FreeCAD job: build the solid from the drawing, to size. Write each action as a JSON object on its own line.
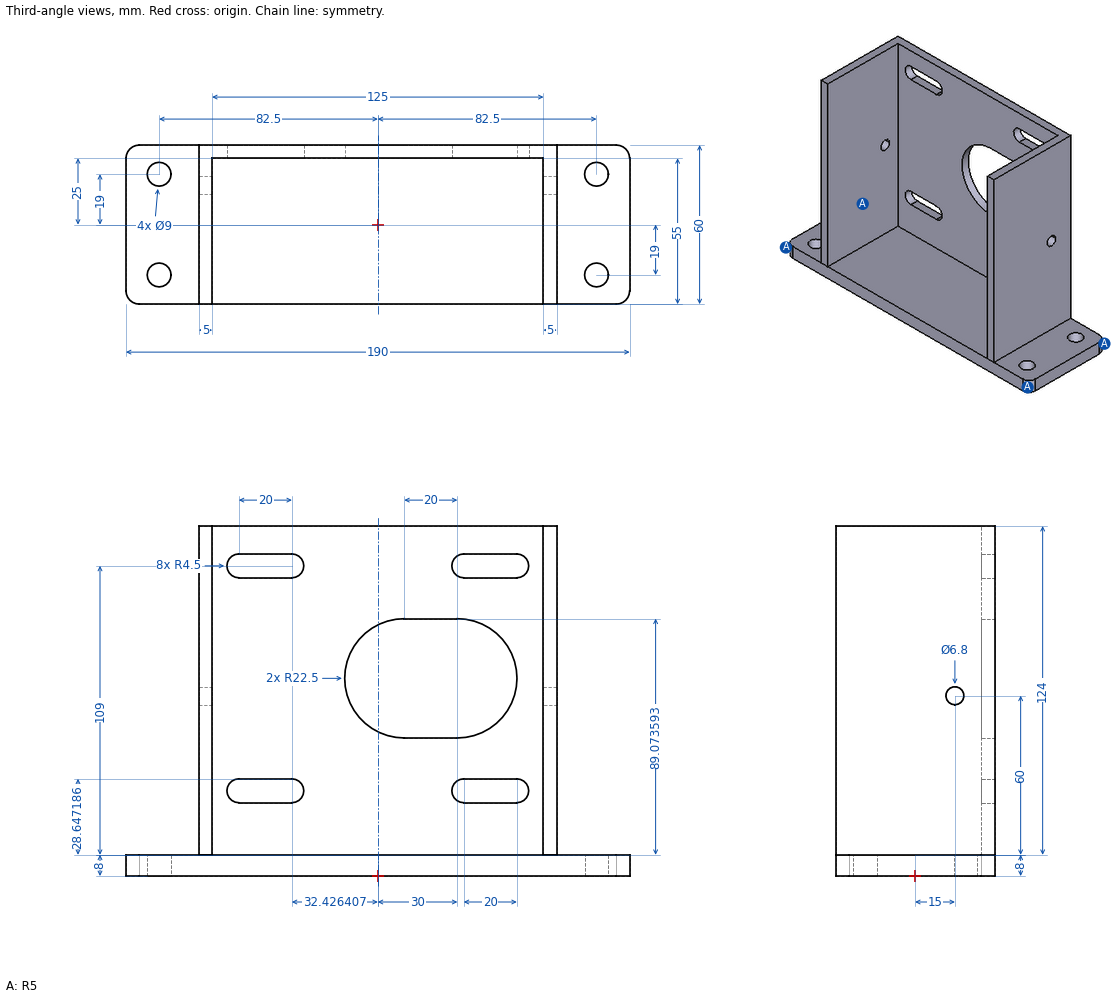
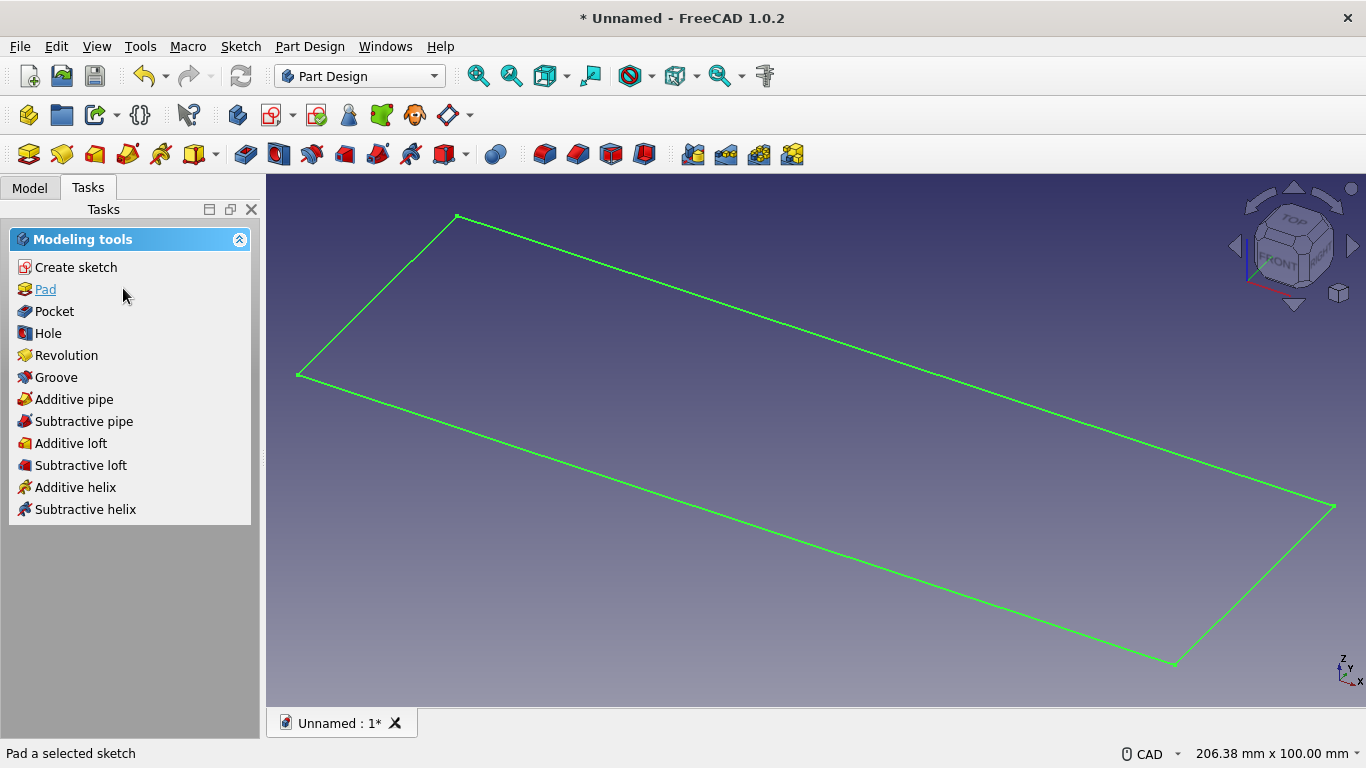
{"action": "left_click", "coordinate": [29, 154]}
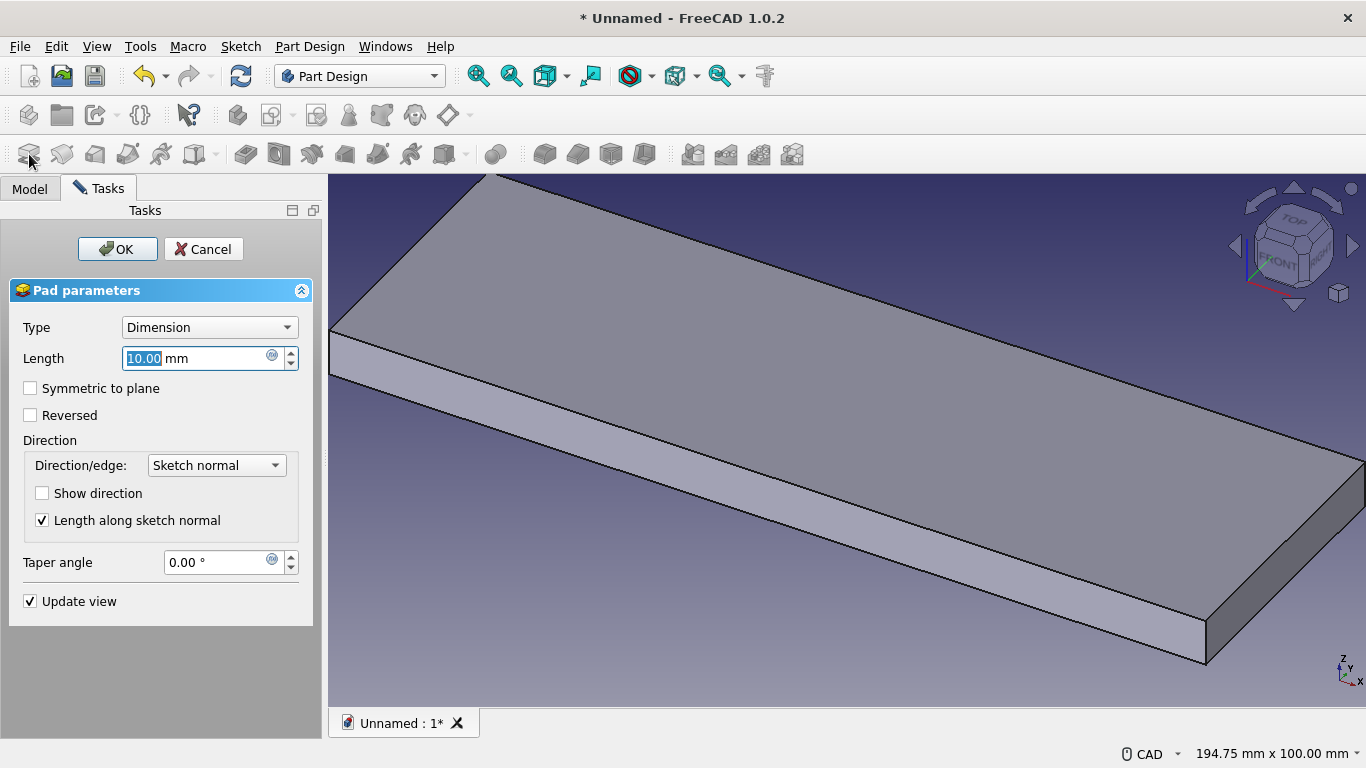
{"action": "type", "text": "8"}
{"action": "key", "text": "Tab"}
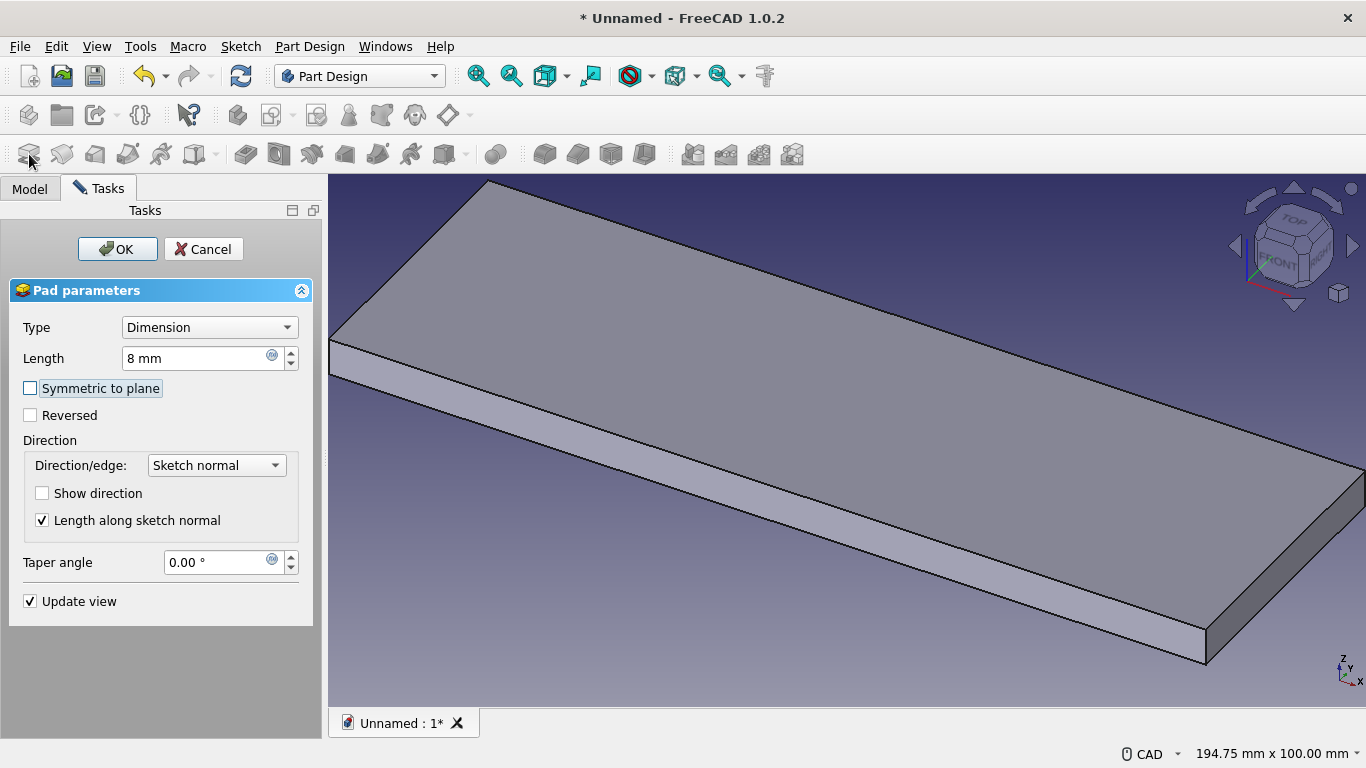
{"action": "left_click", "coordinate": [118, 249]}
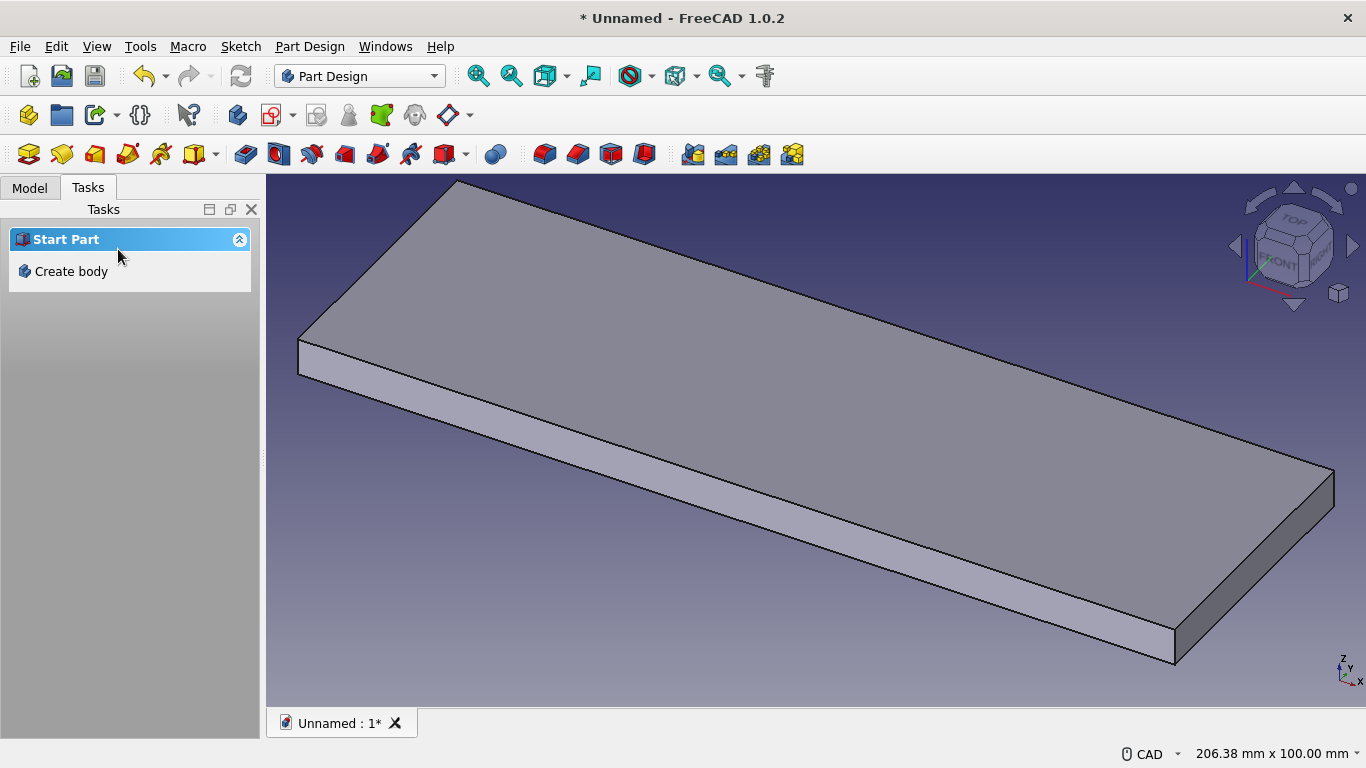
{"action": "left_click", "coordinate": [1067, 487]}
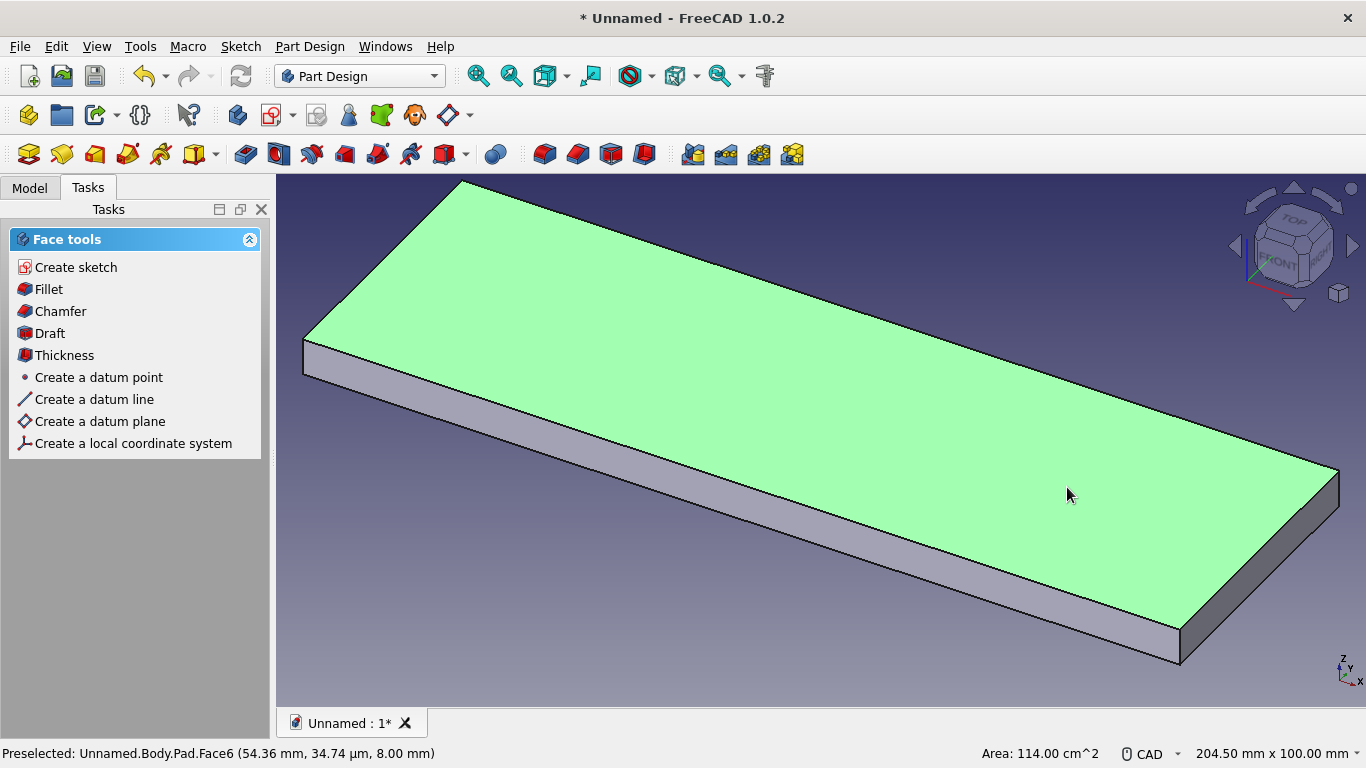
{"action": "left_click", "coordinate": [270, 116]}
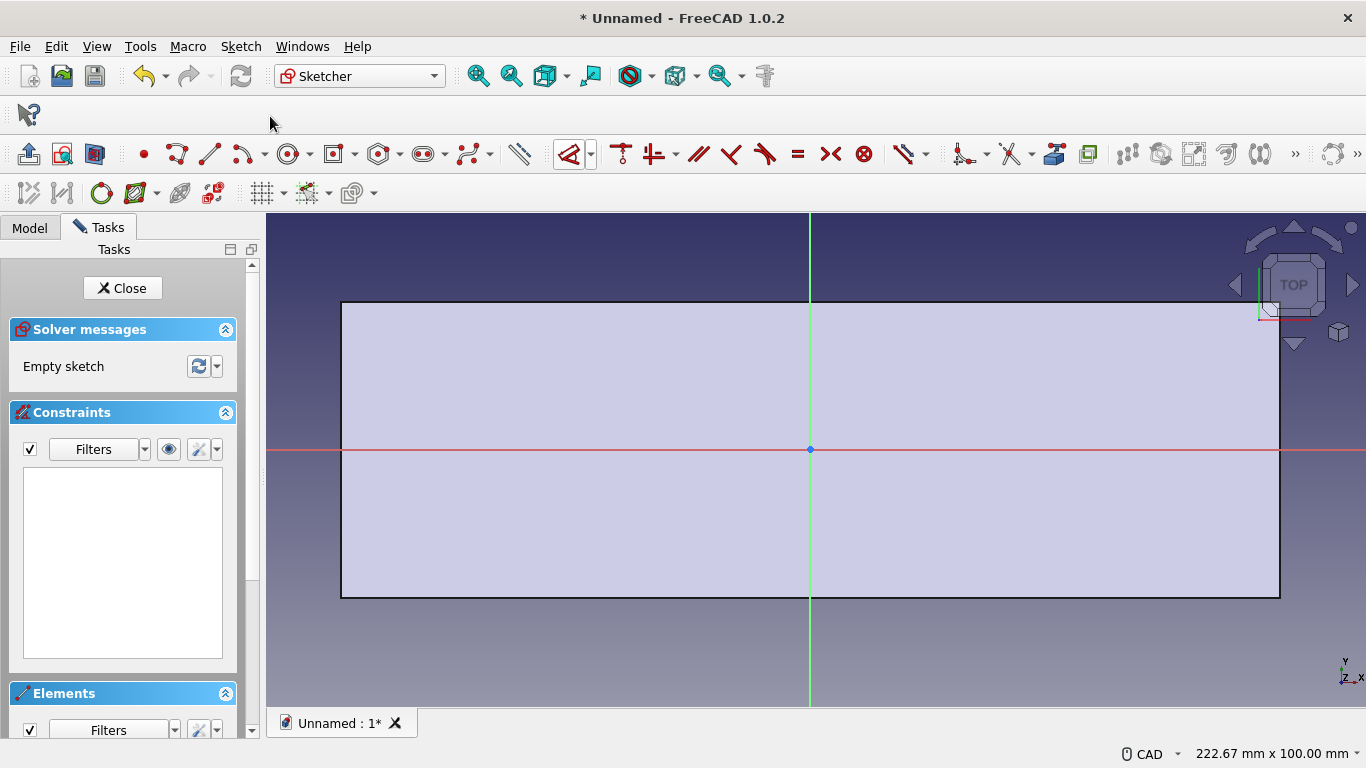
{"action": "scroll", "coordinate": [464, 505], "scroll_direction": "down", "scroll_amount": 1}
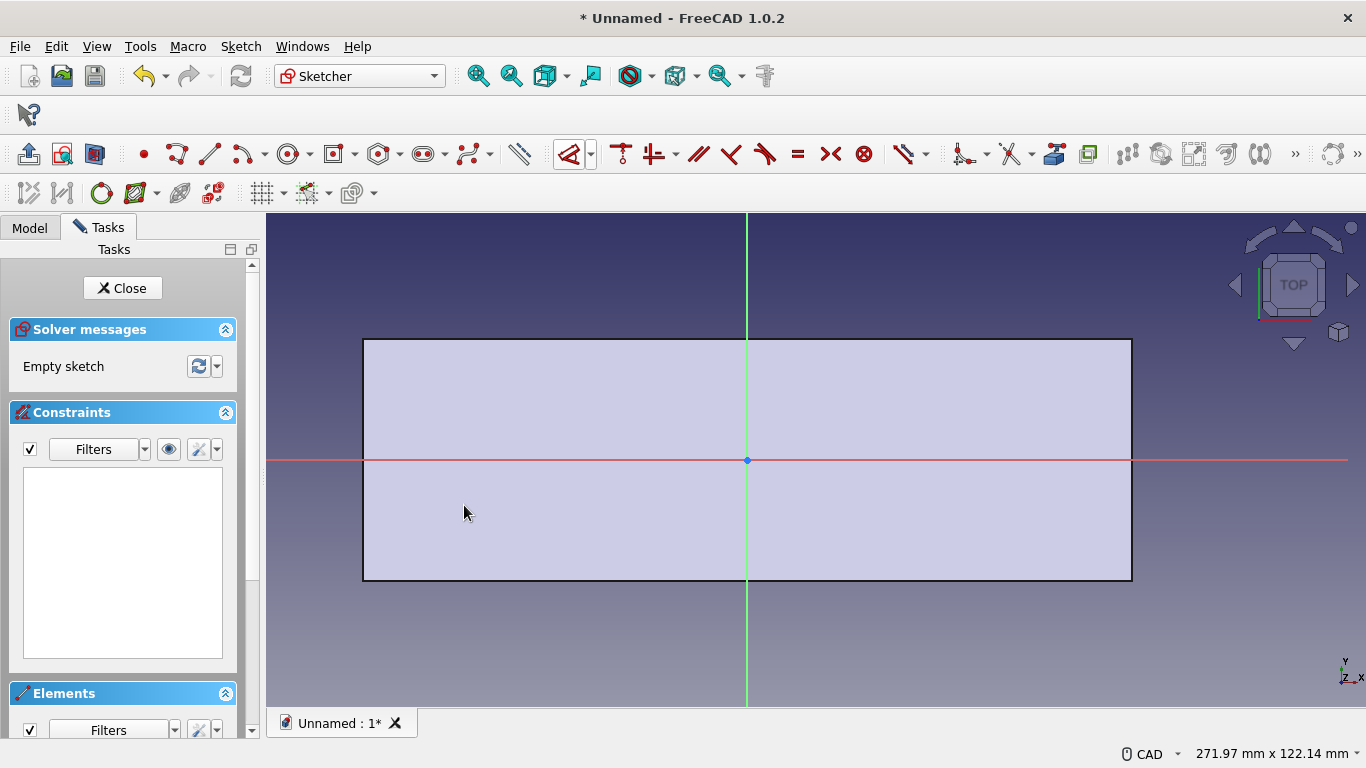
{"action": "left_click", "coordinate": [288, 154]}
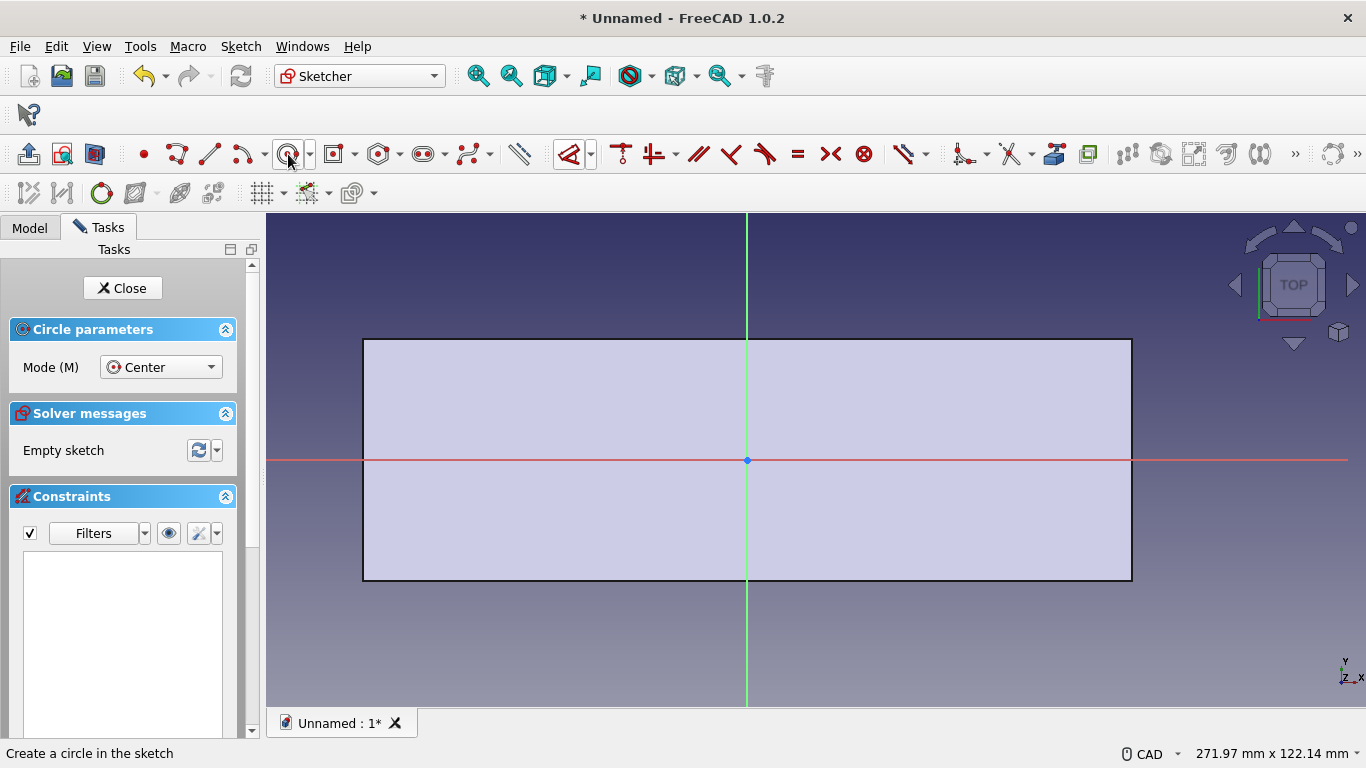
{"action": "scroll", "coordinate": [414, 383], "scroll_direction": "up", "scroll_amount": 2}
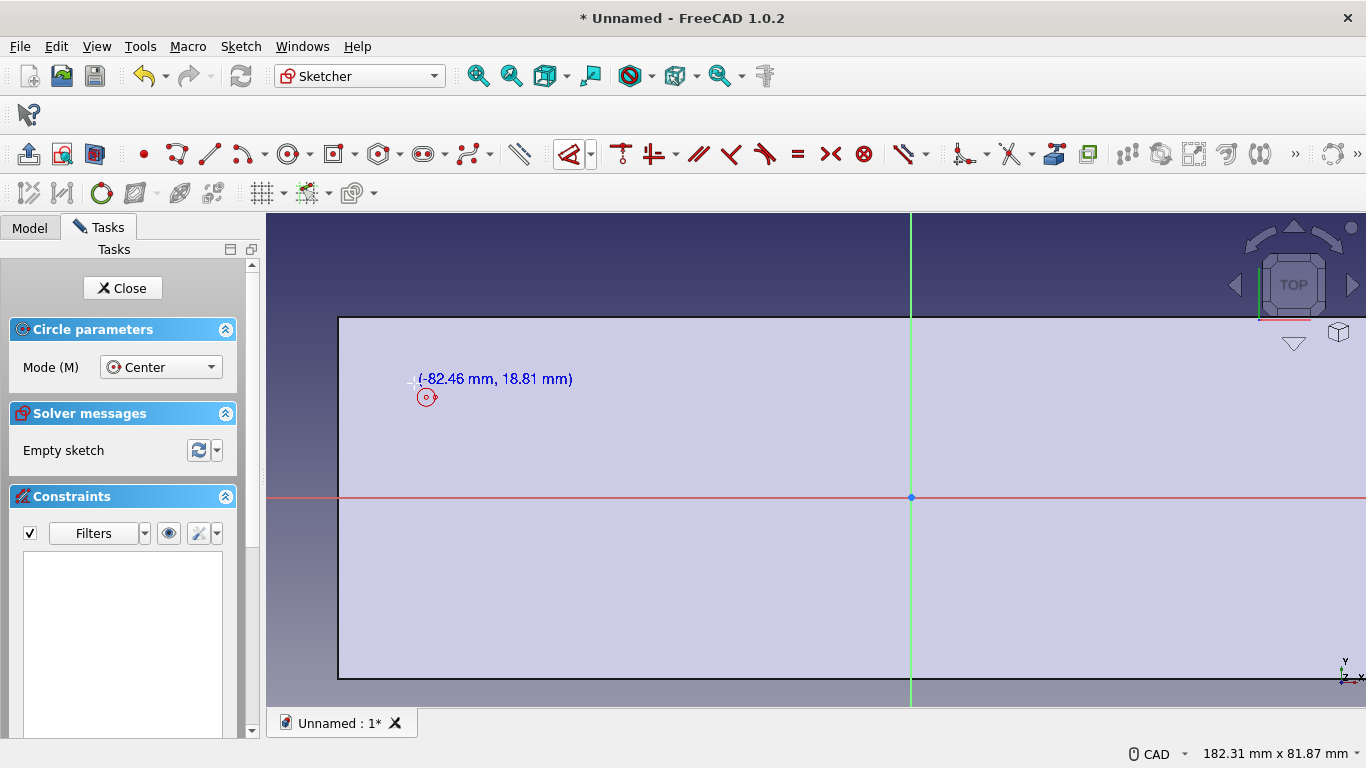
{"action": "left_click", "coordinate": [414, 383]}
{"action": "mouse_move", "coordinate": [433, 364]}